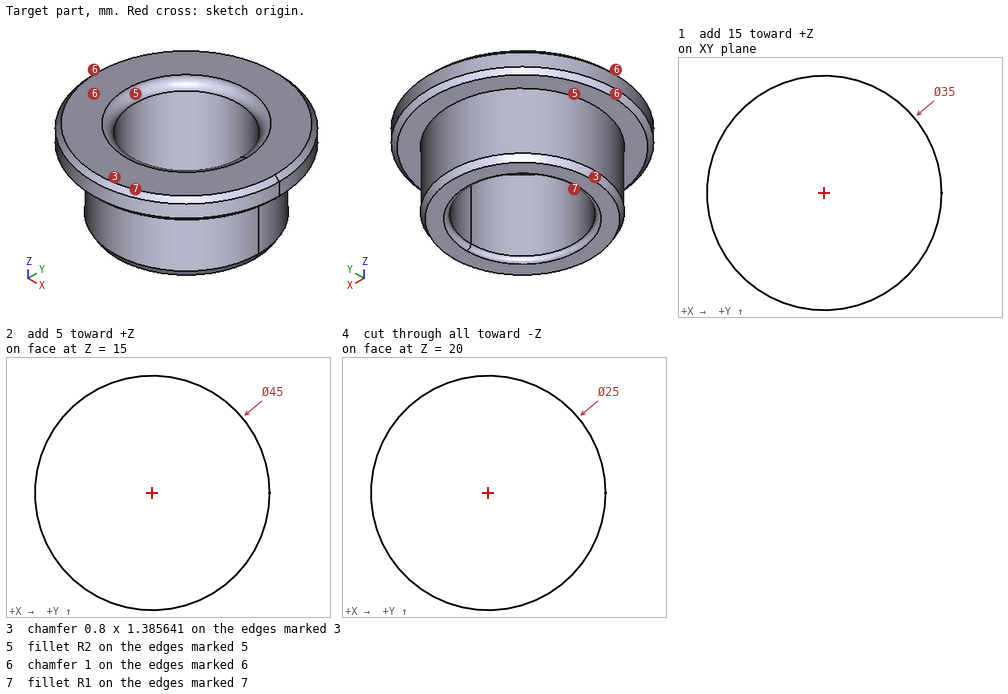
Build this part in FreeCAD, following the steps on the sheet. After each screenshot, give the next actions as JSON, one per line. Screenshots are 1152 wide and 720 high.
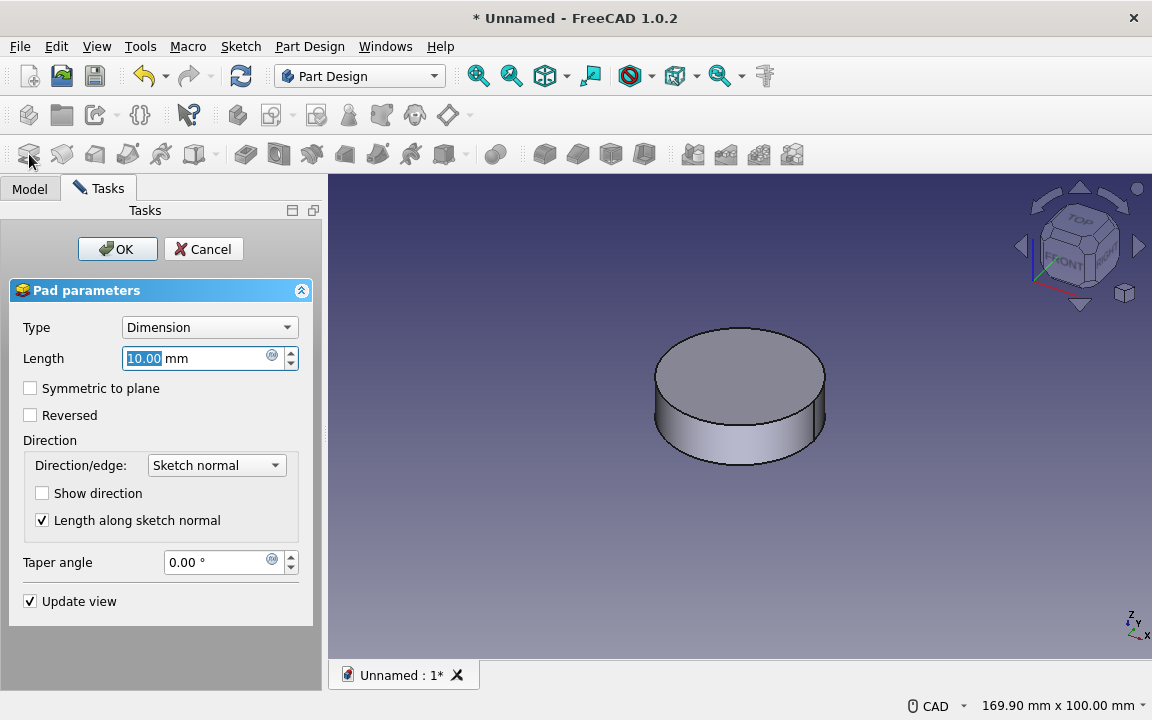
{"action": "type", "text": "15"}
{"action": "key", "text": "Tab"}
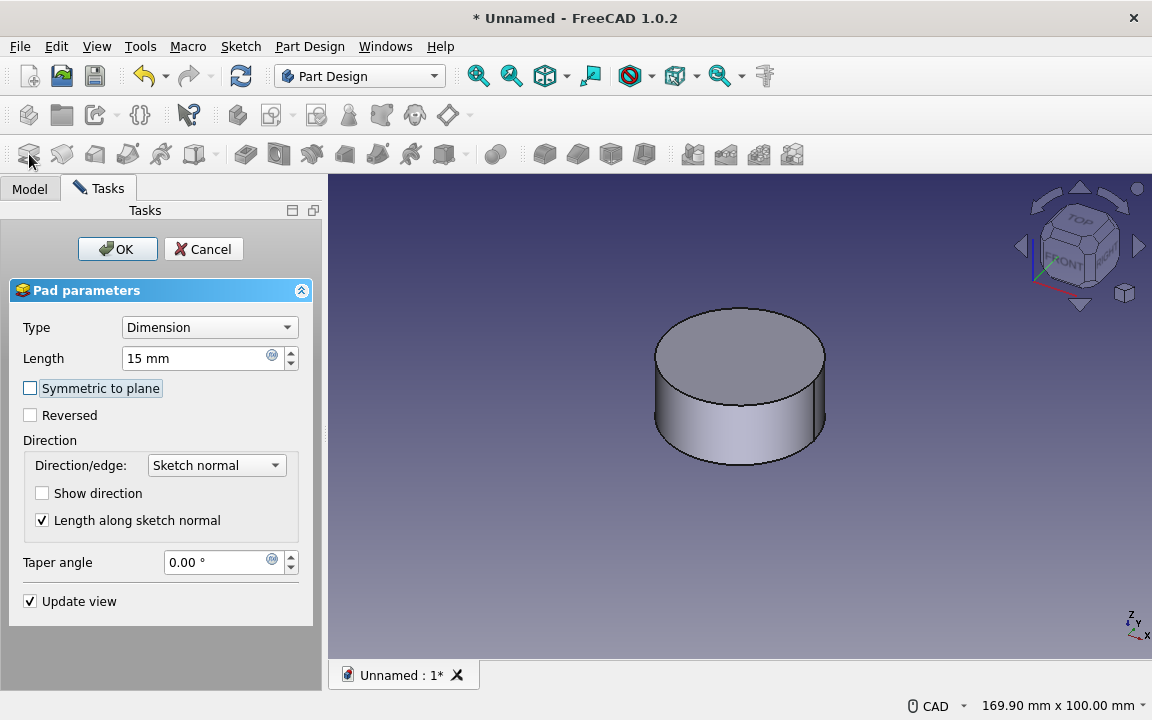
{"action": "left_click", "coordinate": [118, 249]}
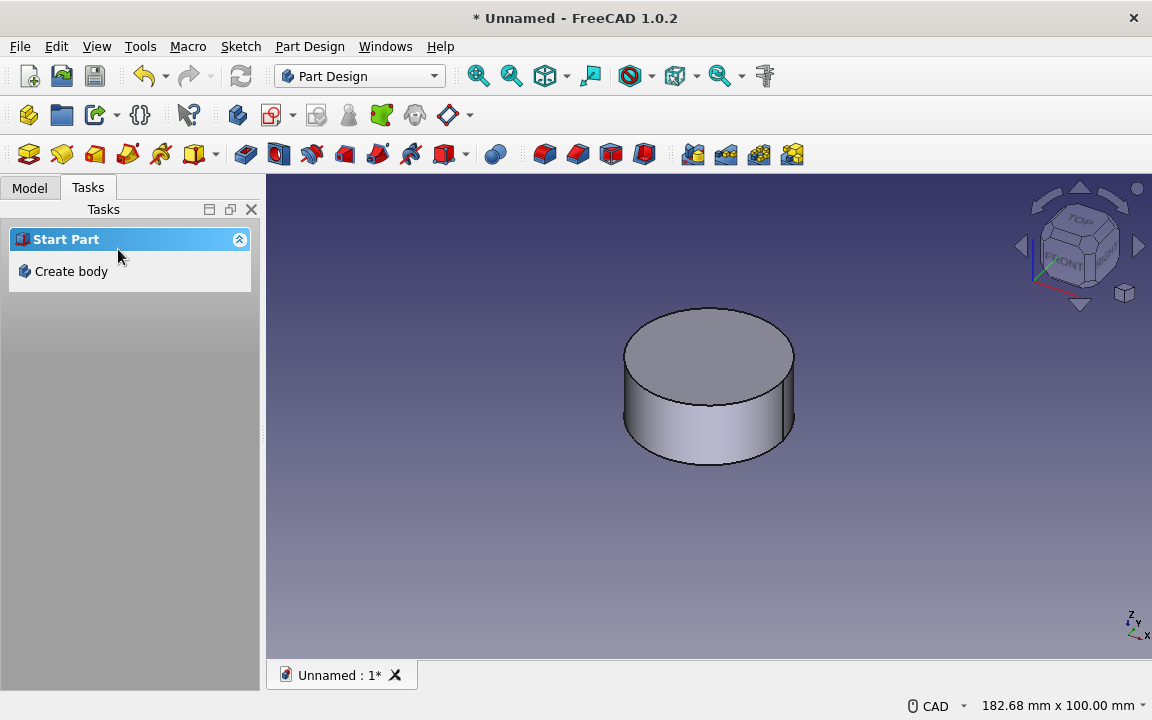
{"action": "left_click", "coordinate": [479, 76]}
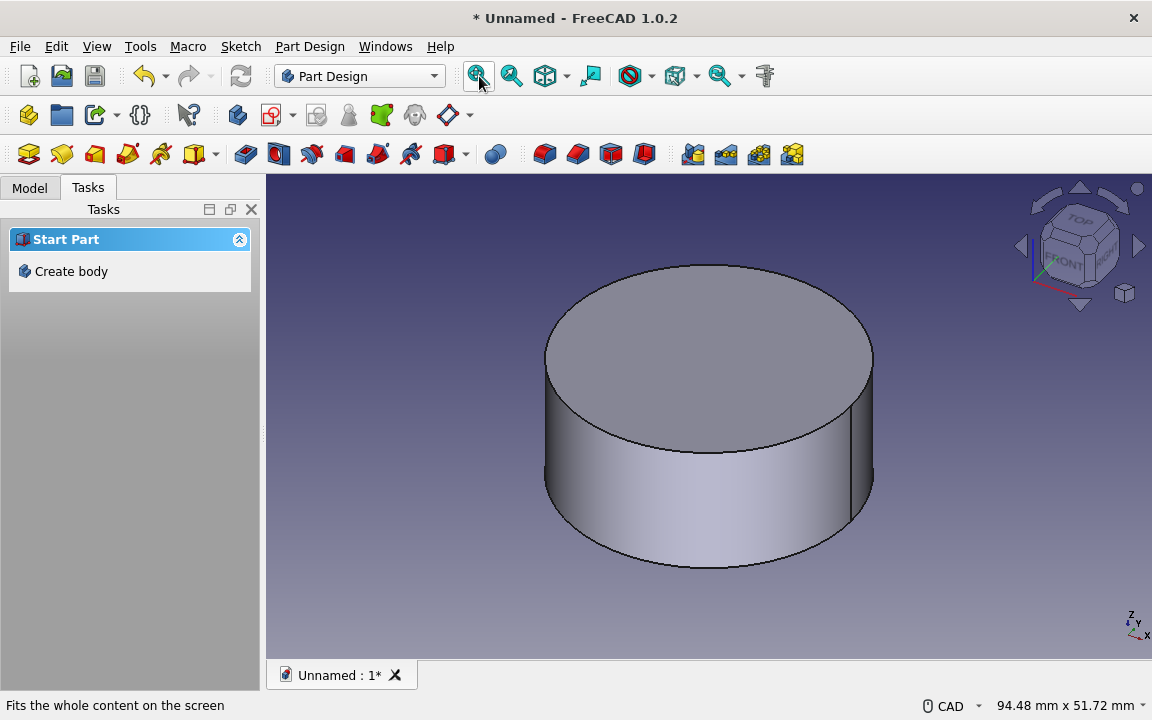
{"action": "left_click", "coordinate": [709, 358]}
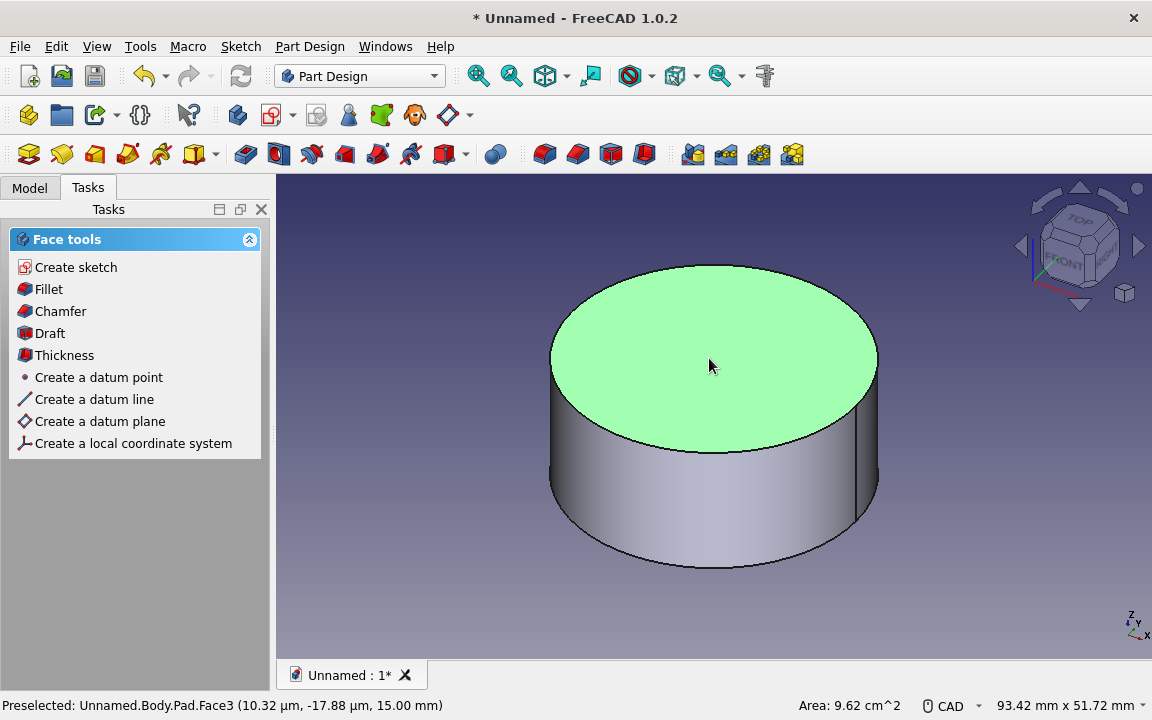
{"action": "left_click", "coordinate": [270, 116]}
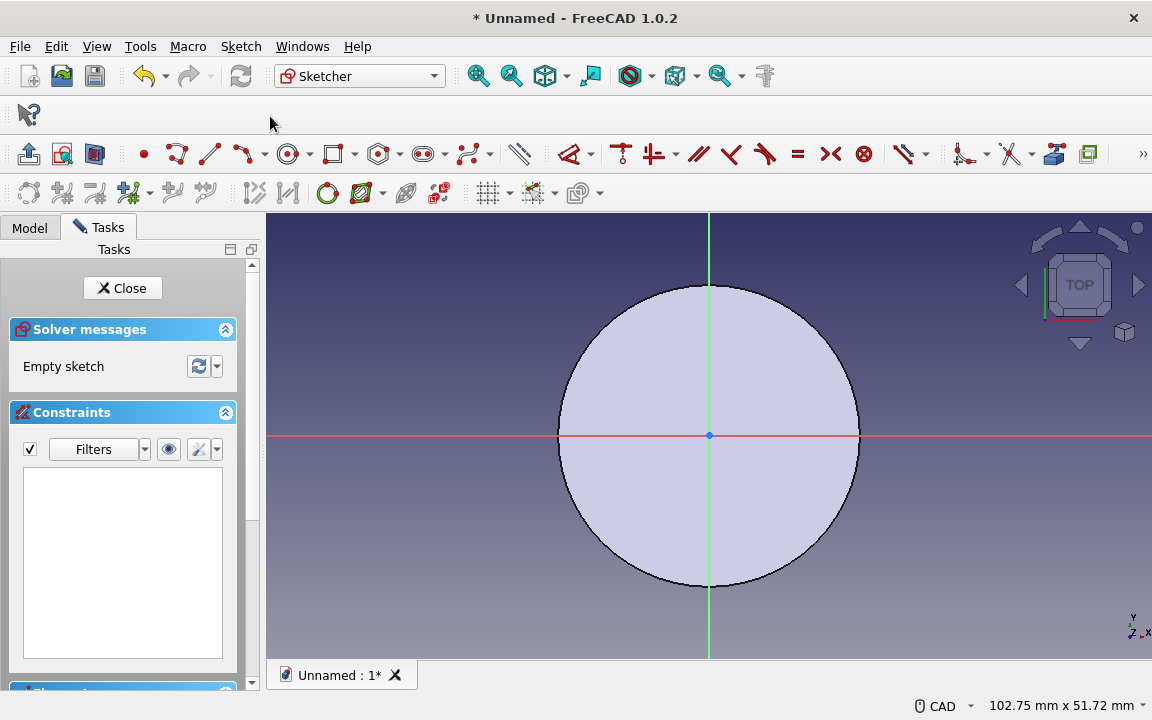
{"action": "scroll", "coordinate": [501, 436], "scroll_direction": "down", "scroll_amount": 2}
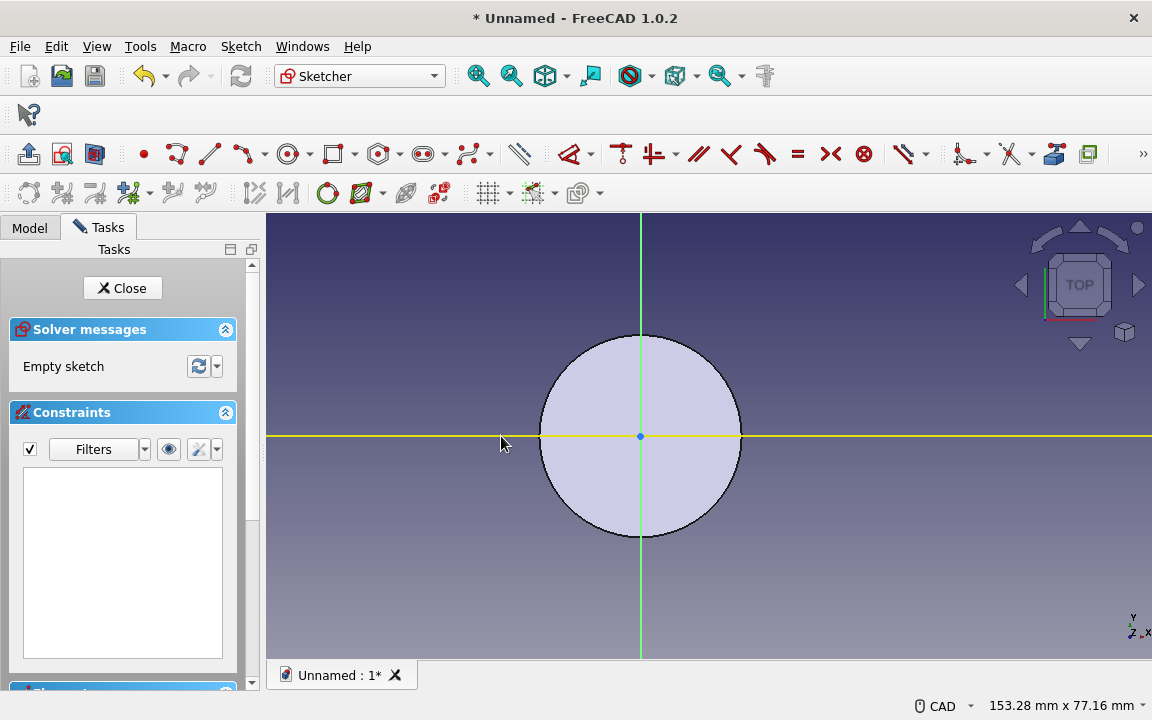
{"action": "key", "text": "g c"}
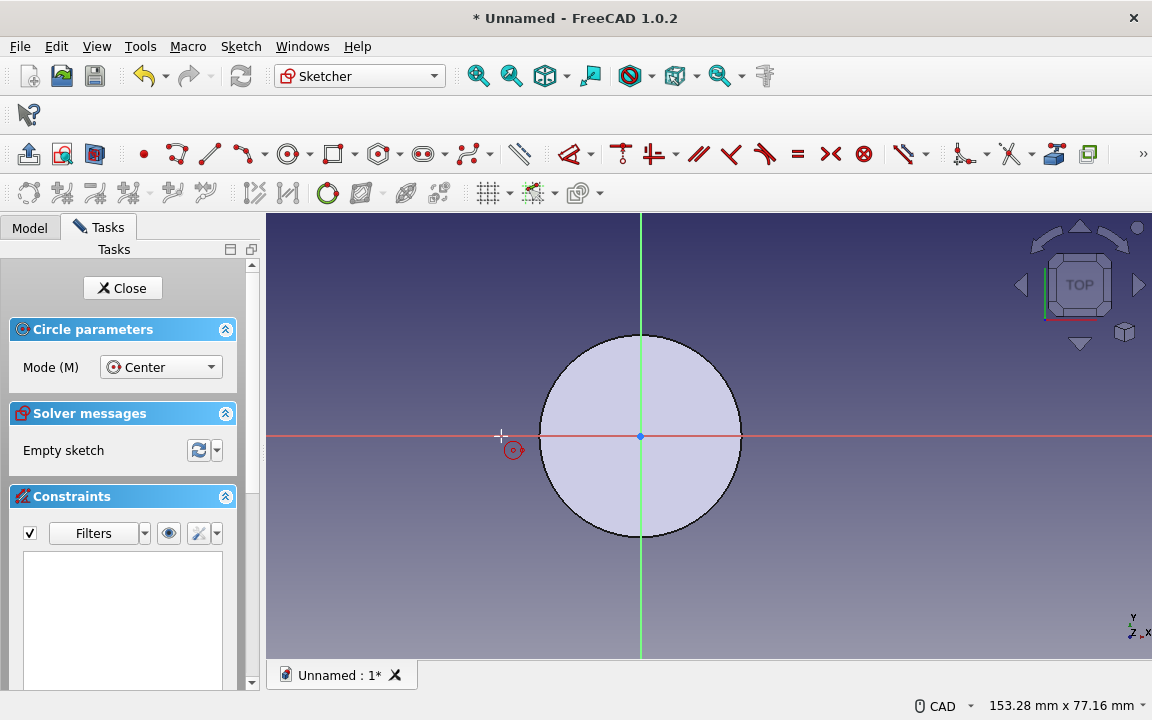
{"action": "left_click", "coordinate": [641, 436]}
{"action": "left_click", "coordinate": [732, 344]}
{"action": "key", "text": "Escape"}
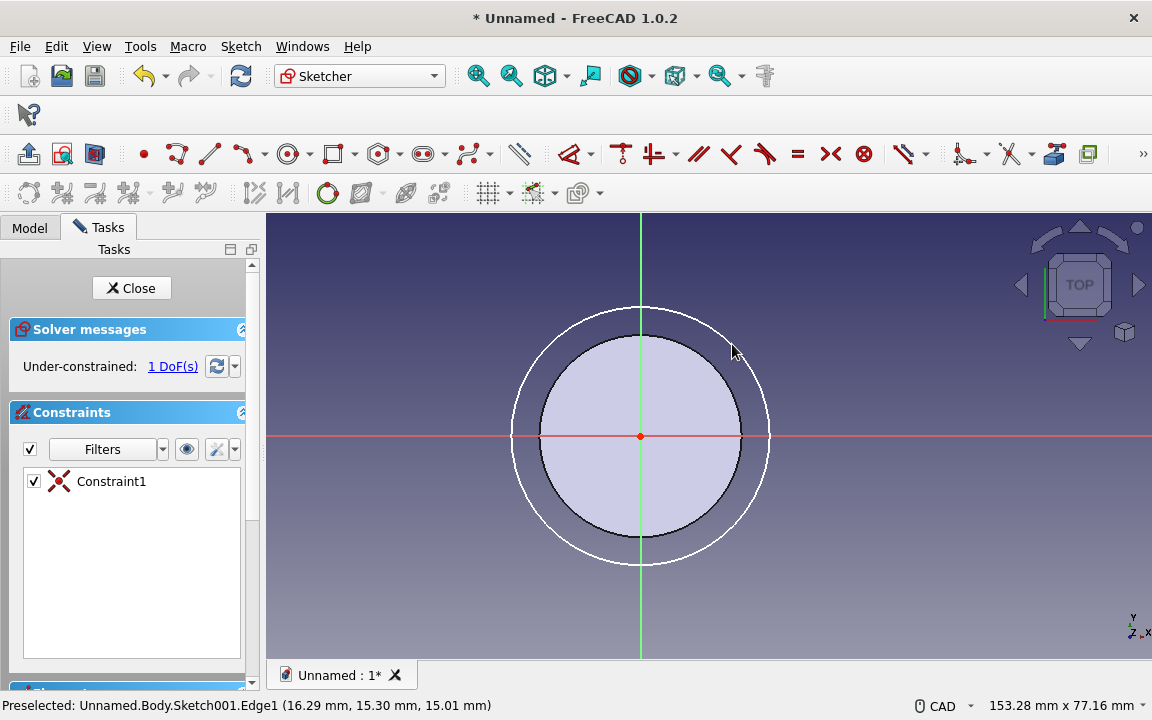
{"action": "left_click", "coordinate": [568, 154]}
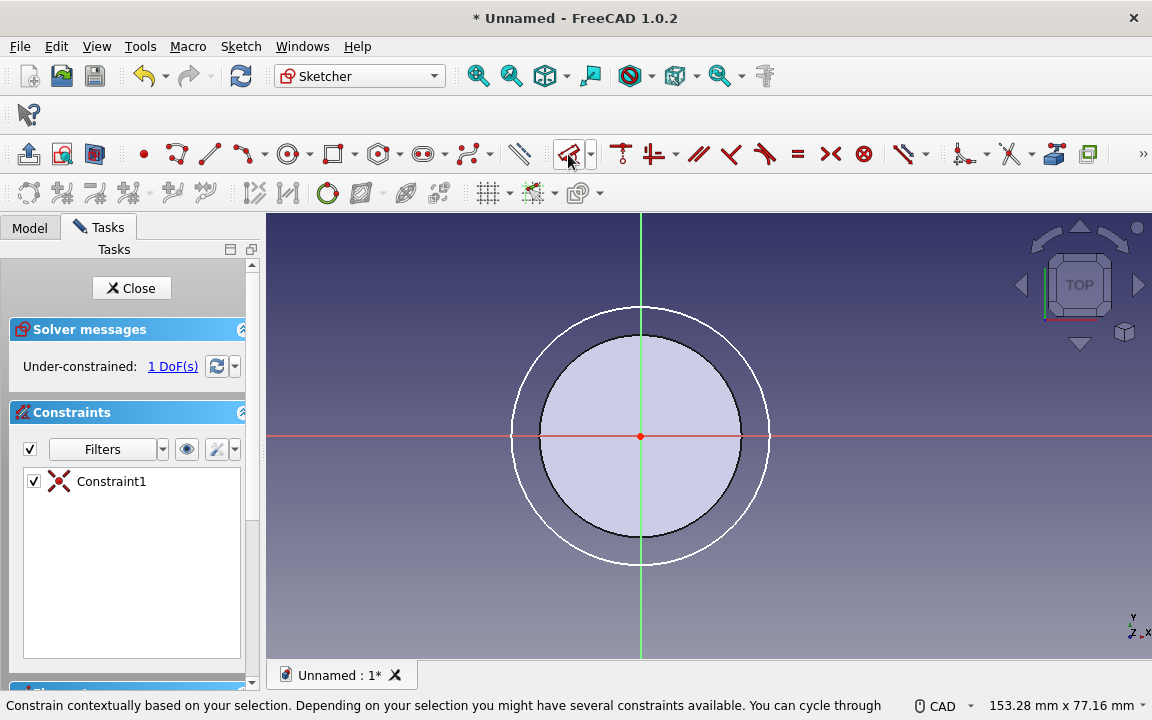
{"action": "left_click", "coordinate": [732, 345]}
{"action": "left_click", "coordinate": [755, 322]}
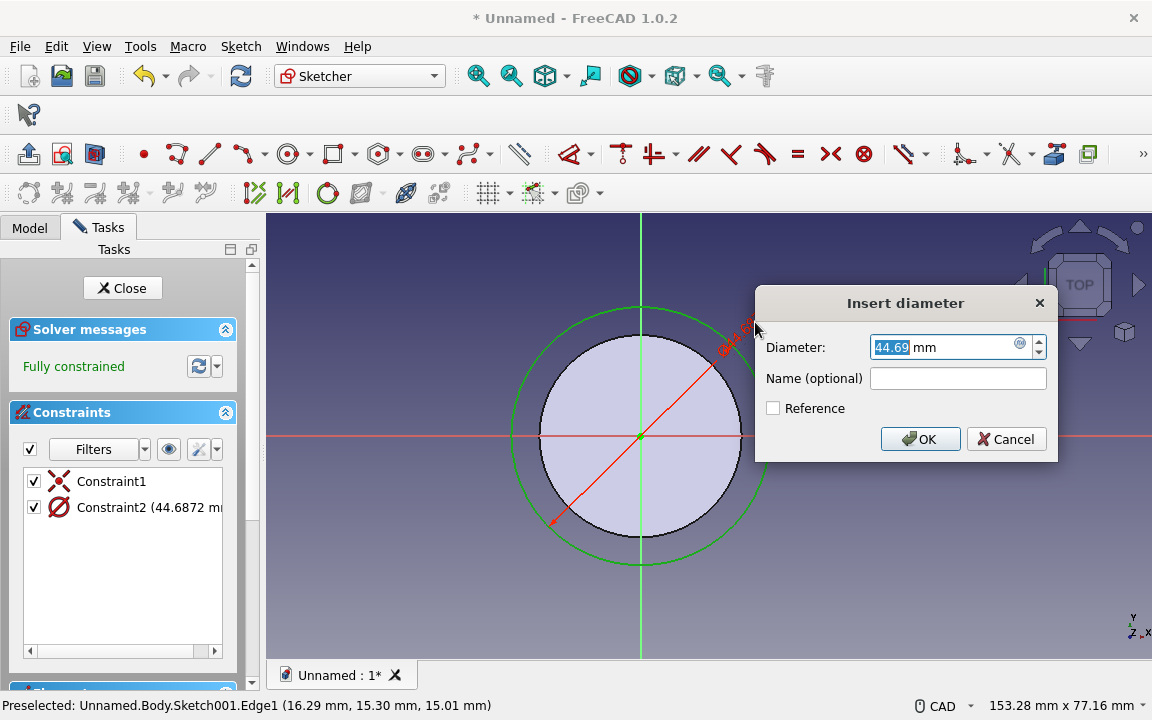
{"action": "type", "text": "45"}
{"action": "key", "text": "Return"}
{"action": "key", "text": "Escape"}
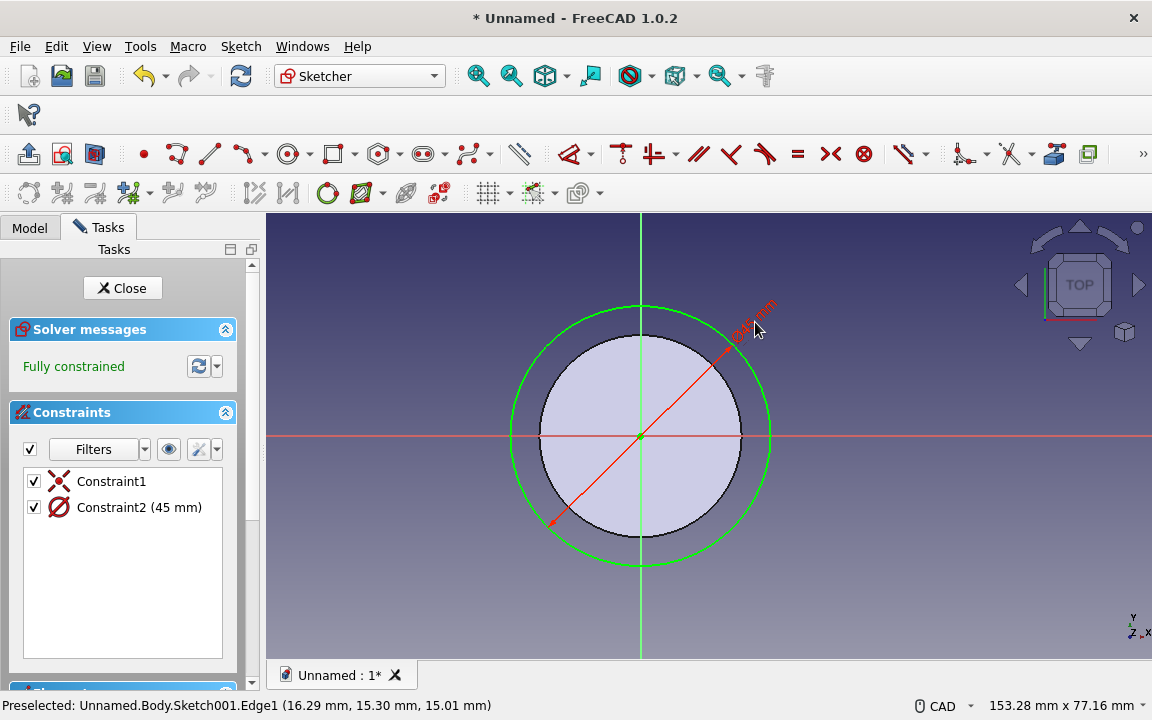
{"action": "left_click", "coordinate": [123, 288]}